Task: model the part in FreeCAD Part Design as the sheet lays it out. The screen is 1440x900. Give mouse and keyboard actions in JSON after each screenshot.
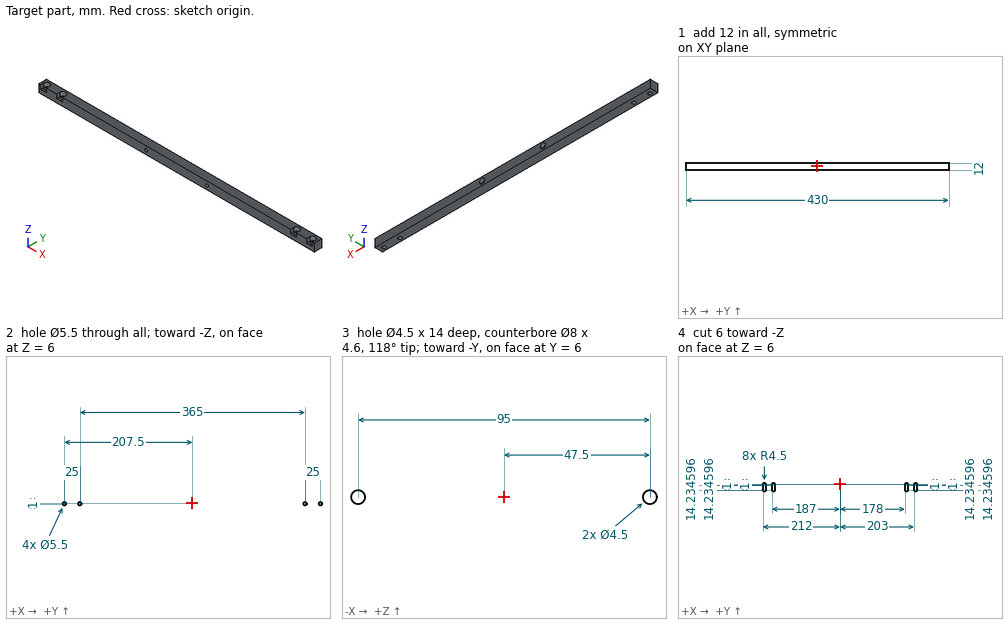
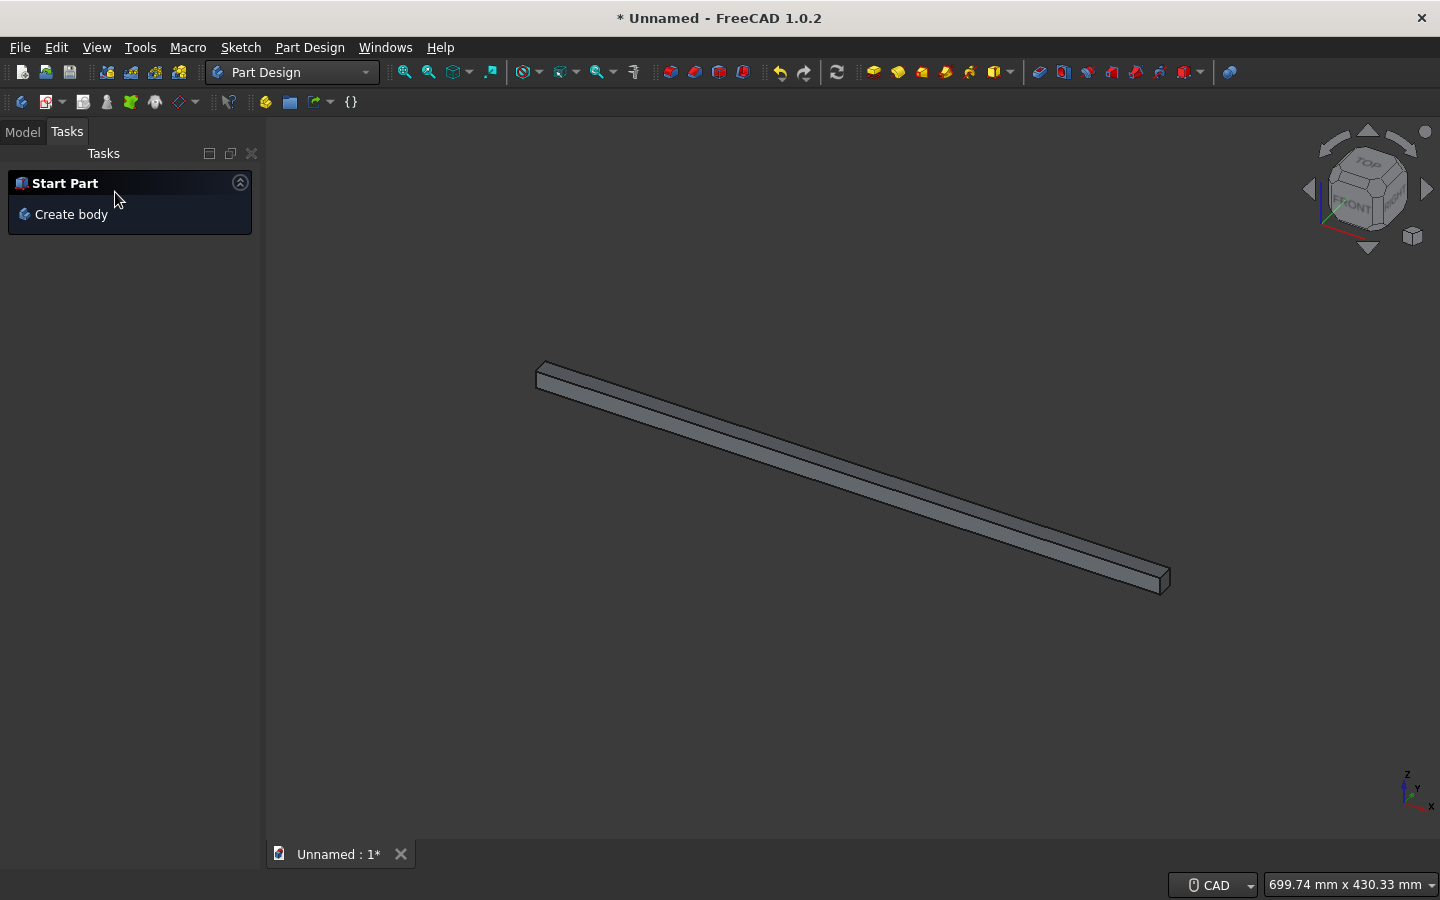
{"action": "key", "text": "0"}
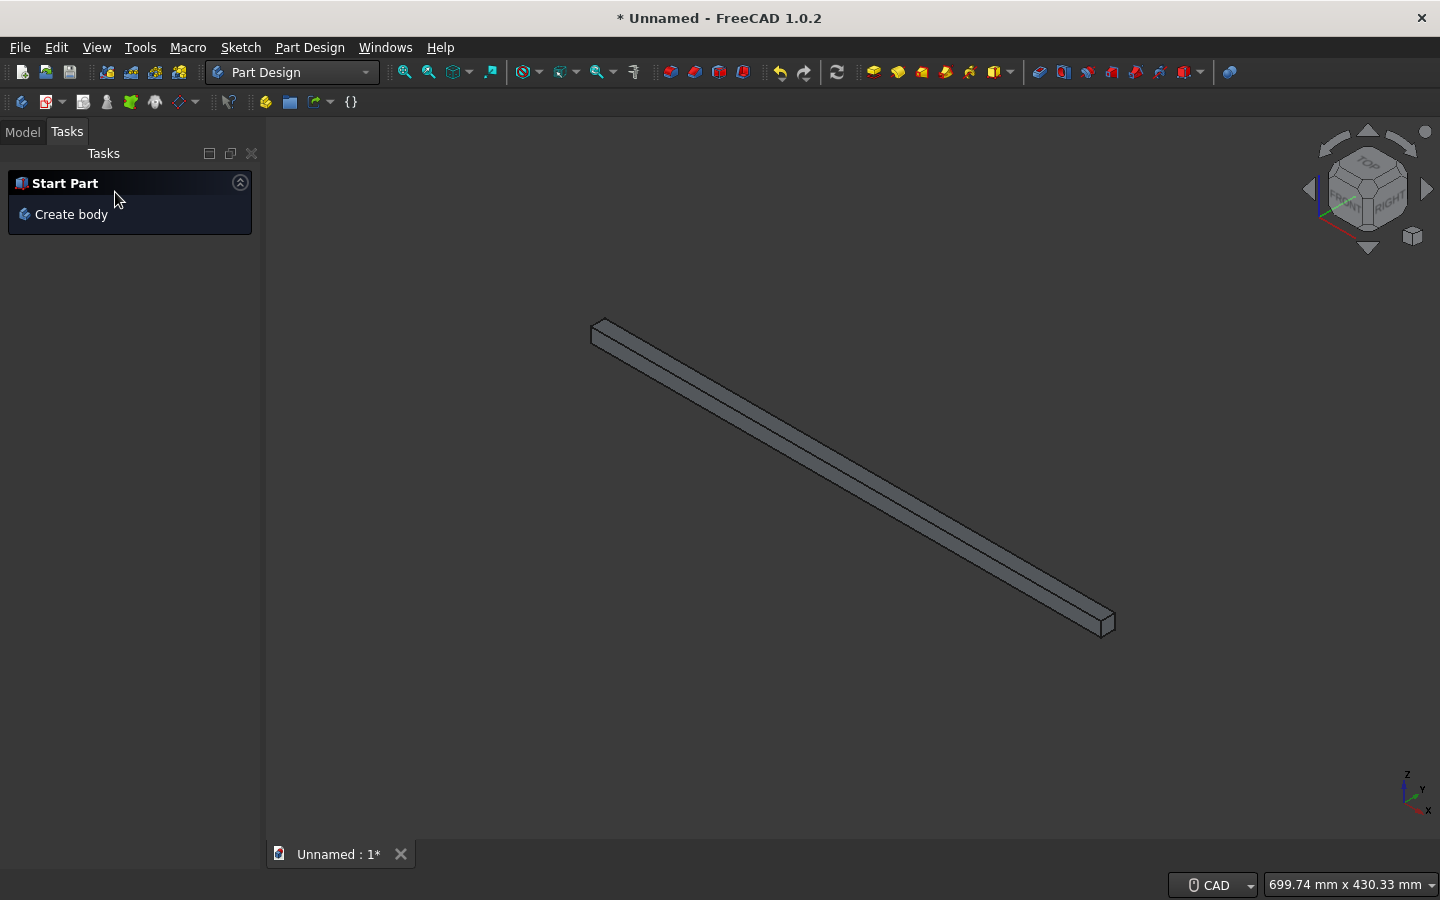
{"action": "left_click", "coordinate": [406, 72]}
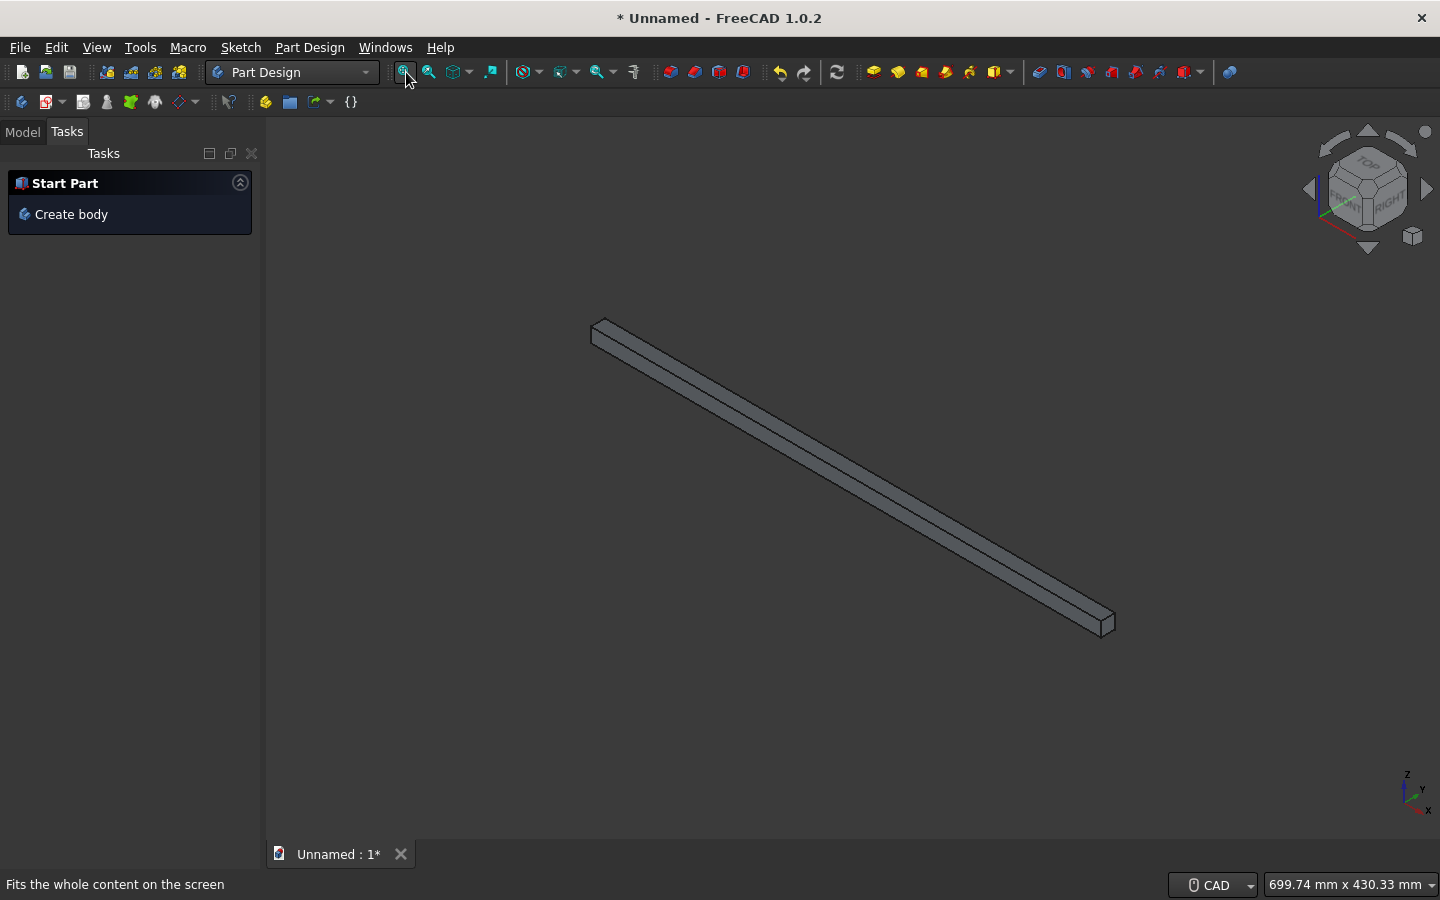
{"action": "left_click", "coordinate": [1074, 594]}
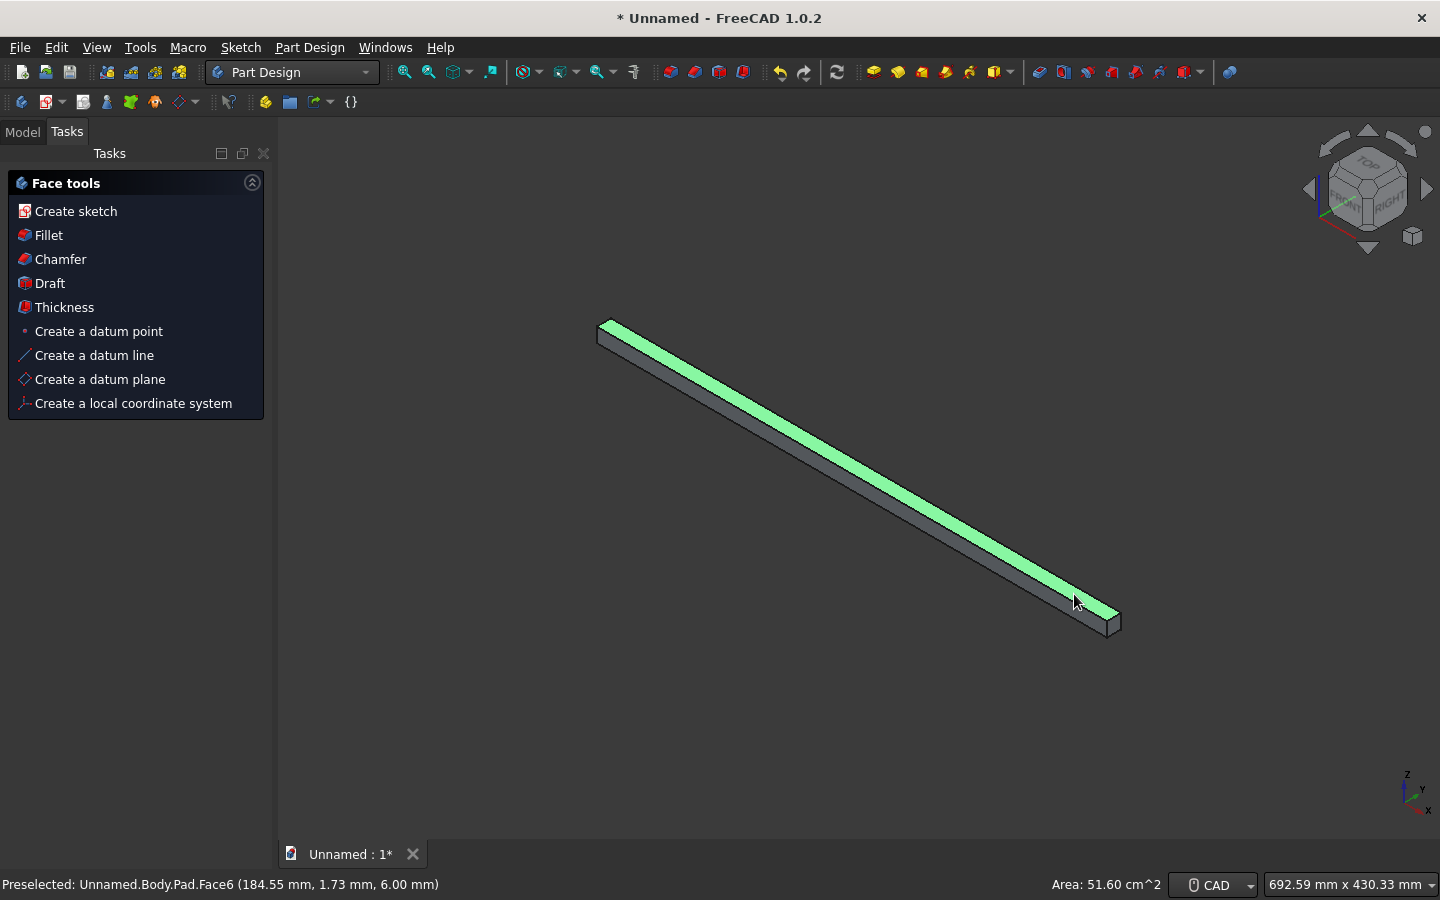
{"action": "left_click", "coordinate": [46, 102]}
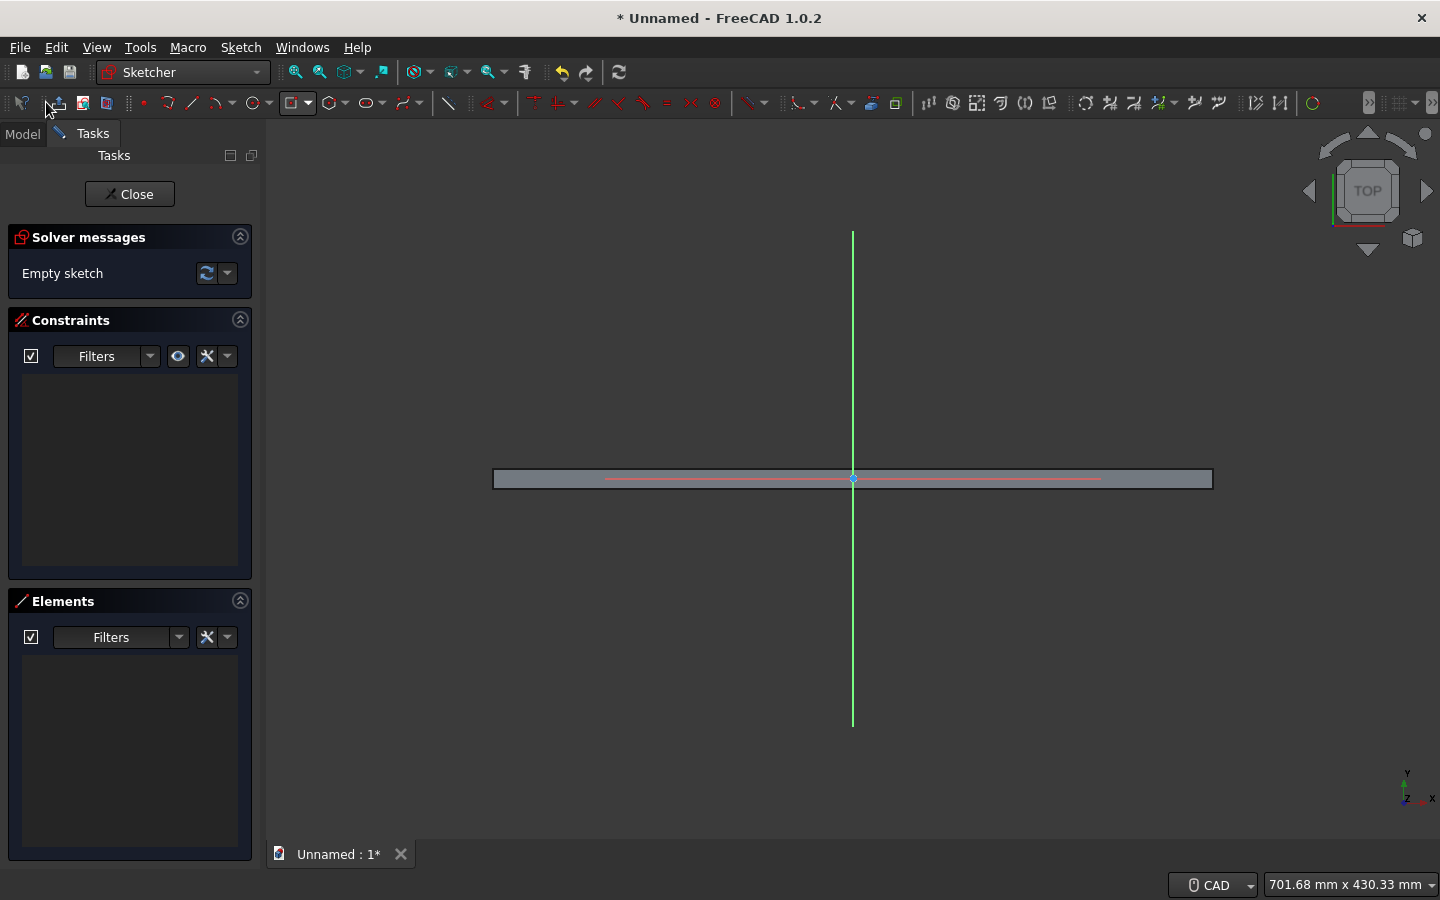
{"action": "left_click", "coordinate": [254, 104]}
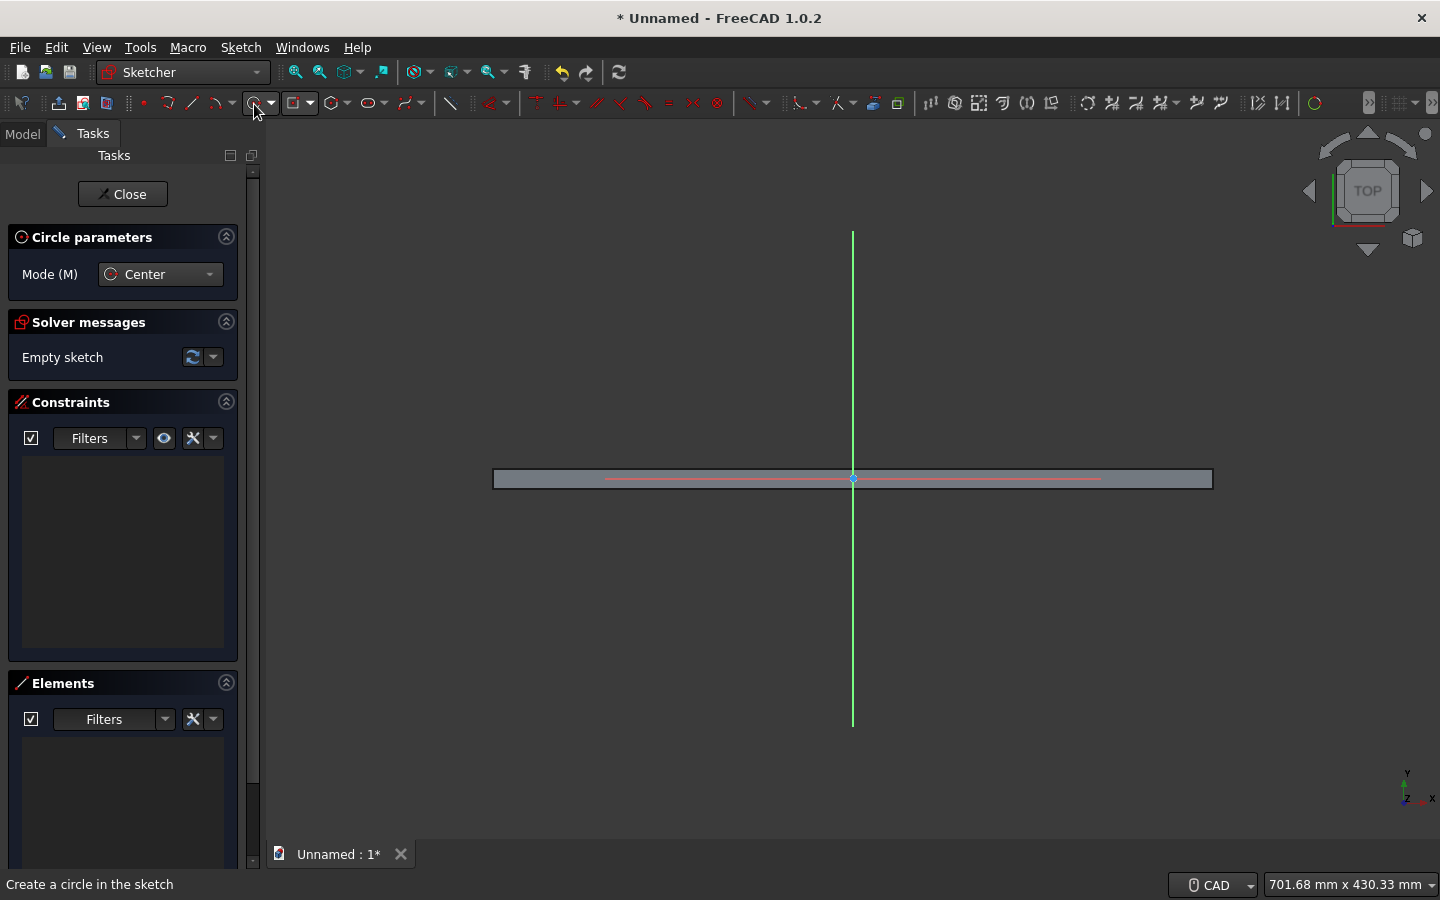
{"action": "scroll", "coordinate": [506, 481], "scroll_direction": "up", "scroll_amount": 12}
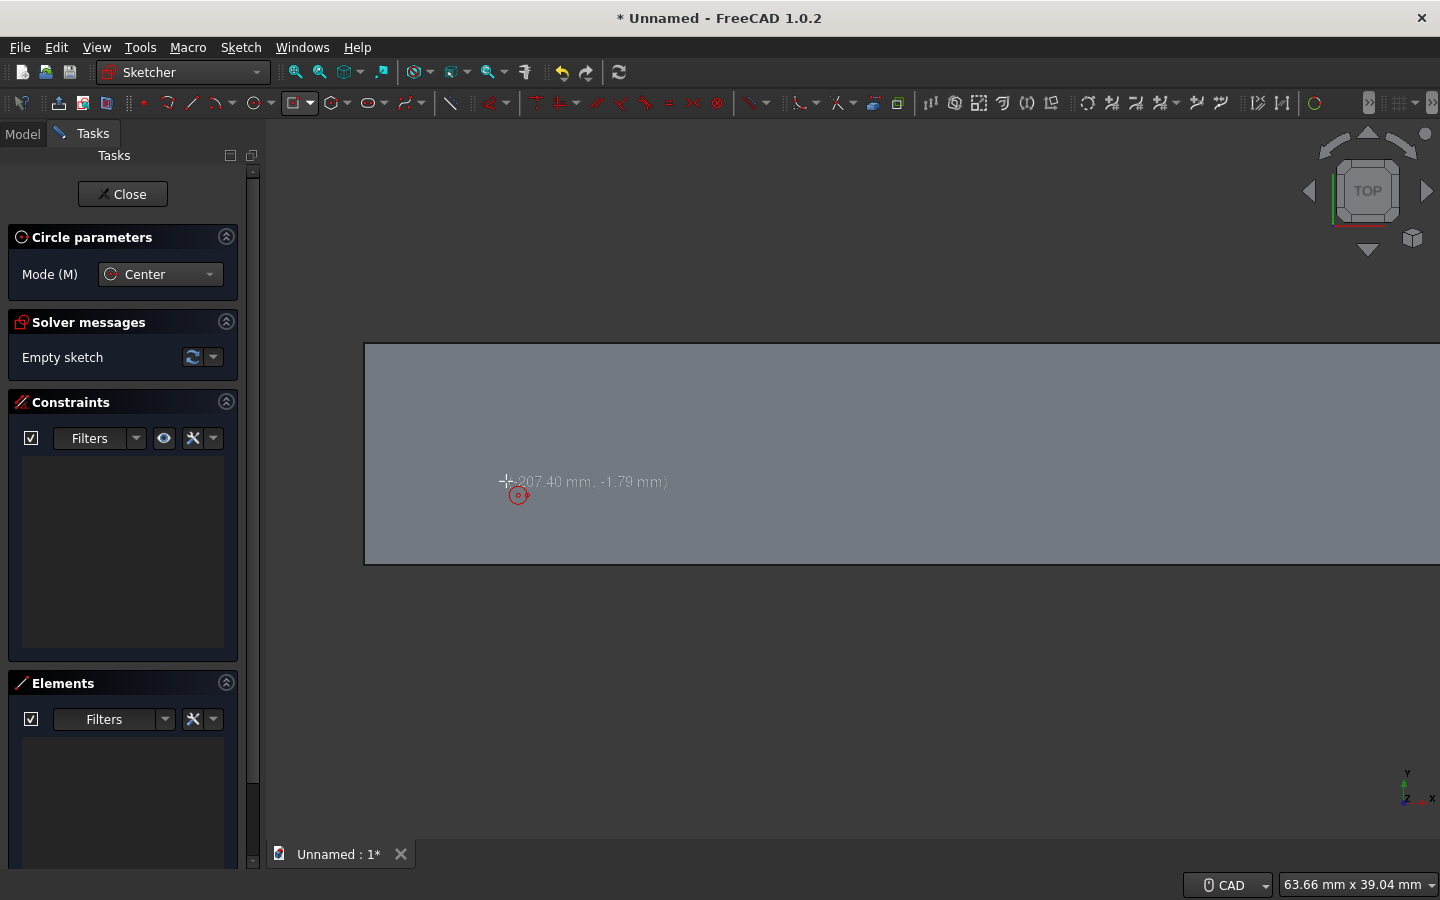
{"action": "left_click", "coordinate": [502, 472]}
{"action": "mouse_move", "coordinate": [538, 436]}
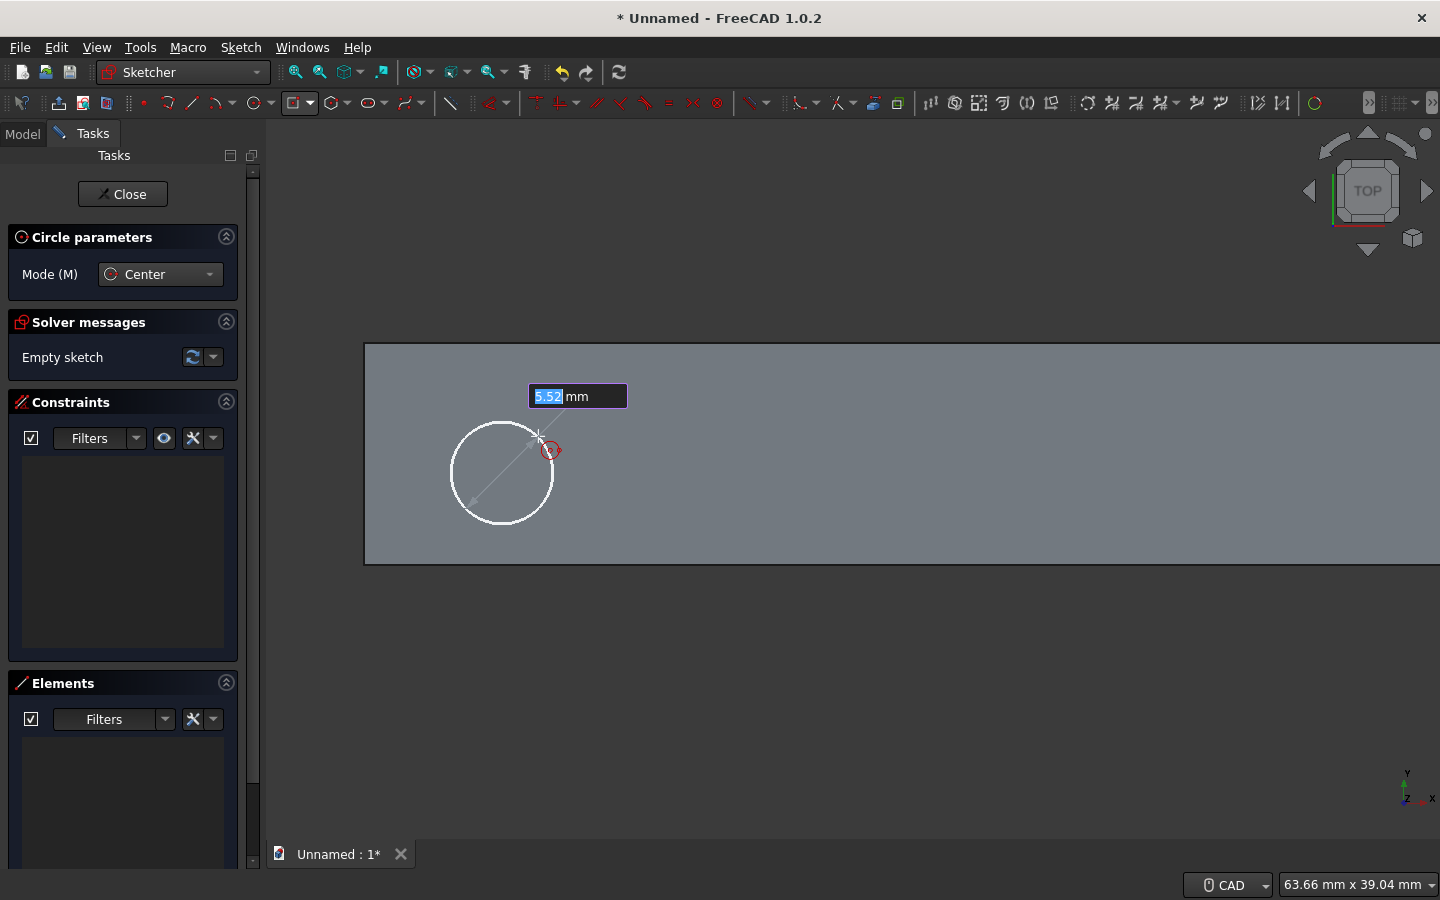
{"action": "type", "text": "5.5"}
{"action": "key", "text": "Return"}